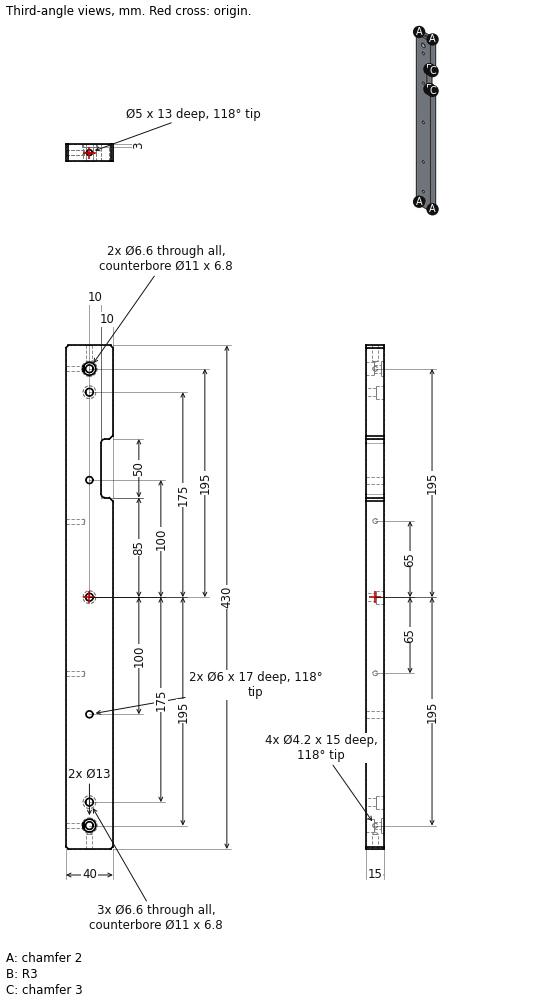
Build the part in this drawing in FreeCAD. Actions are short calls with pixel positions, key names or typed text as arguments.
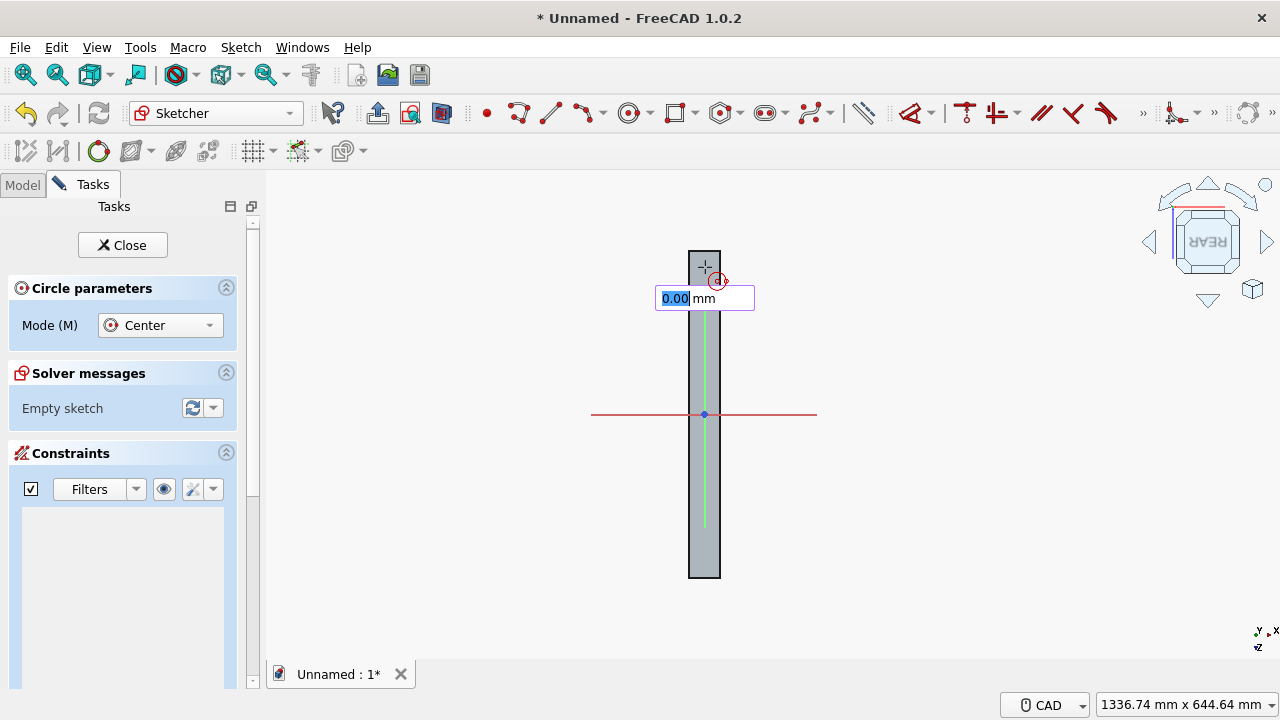
scroll(709, 265, up, 7)
move(708, 264)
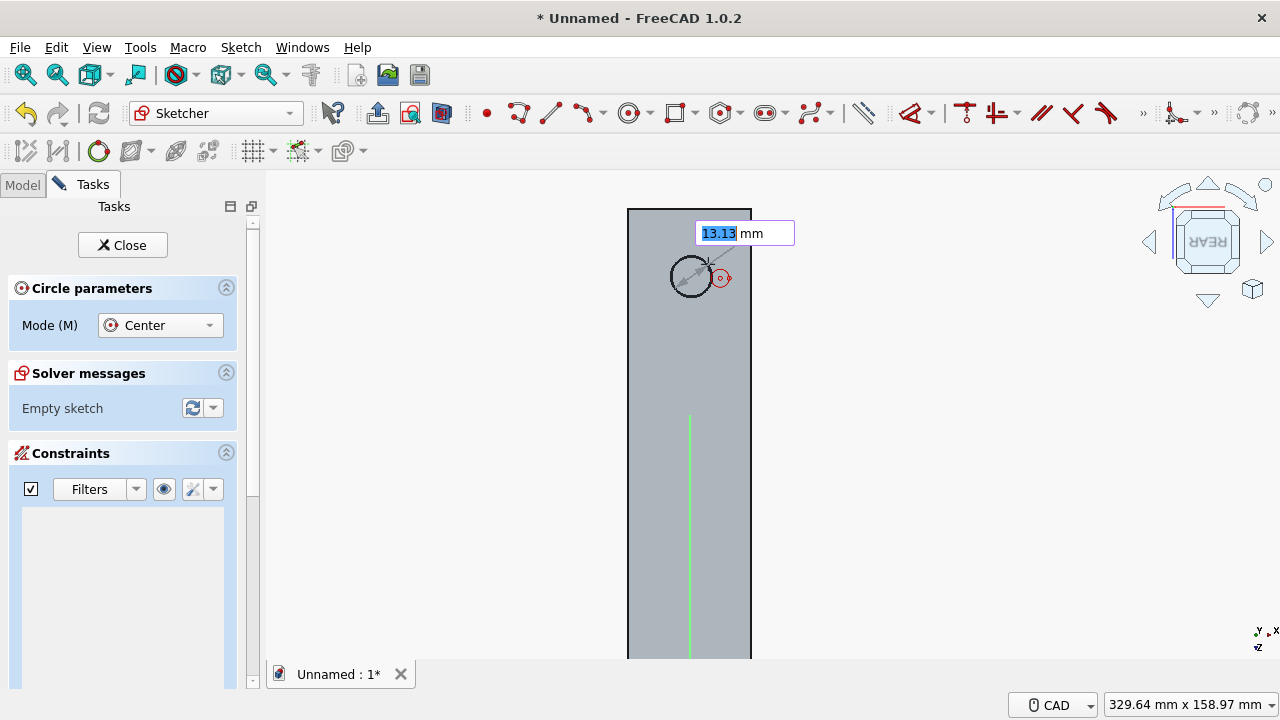
text(13)
key(Return)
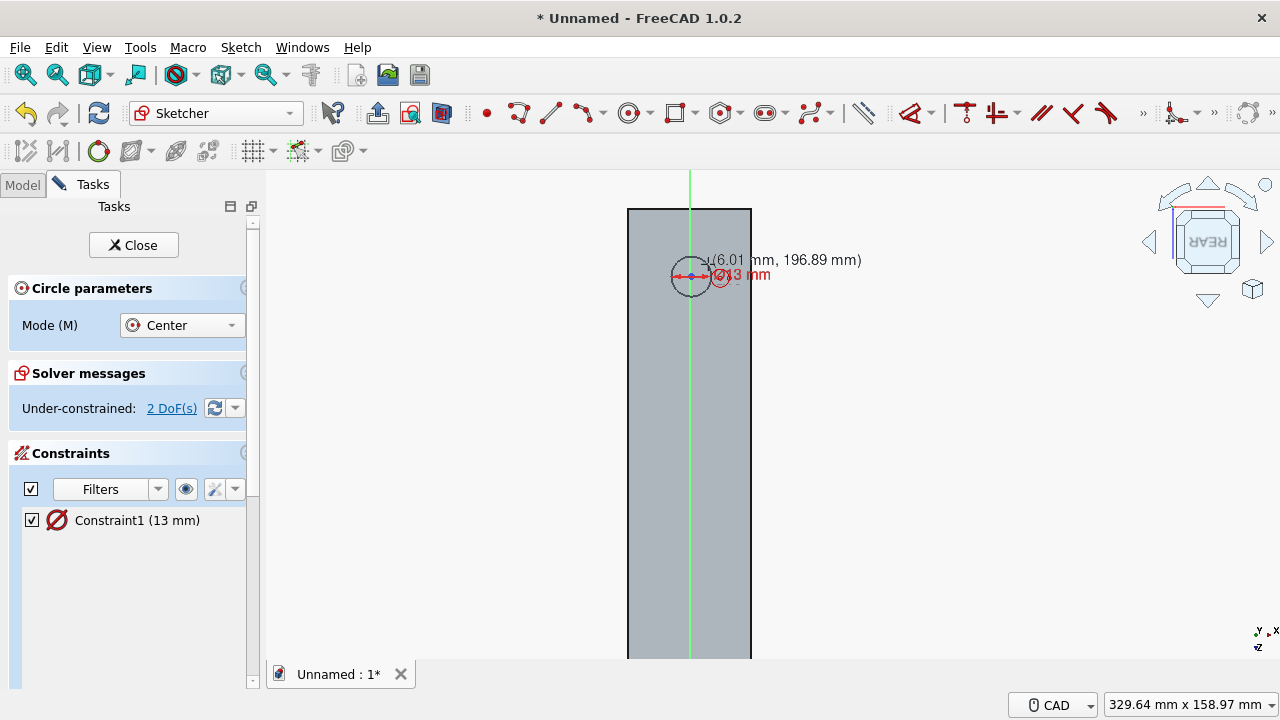
scroll(709, 265, down, 7)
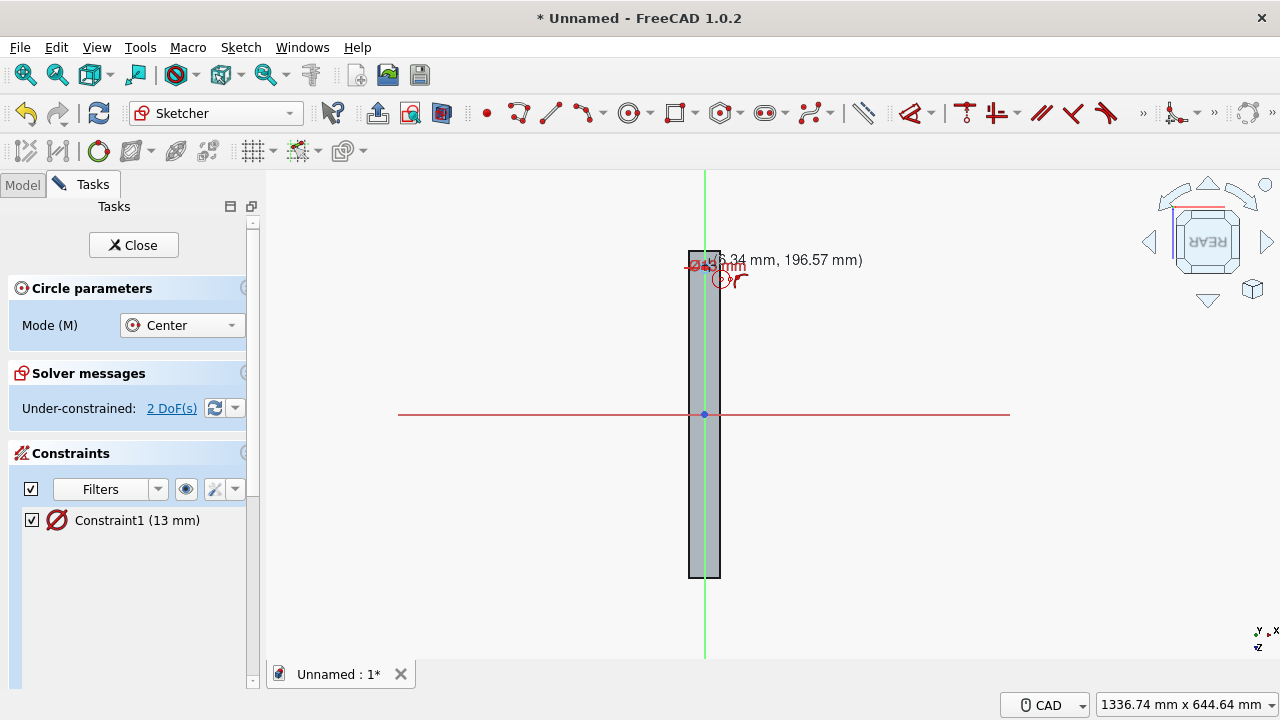
scroll(705, 562, up, 8)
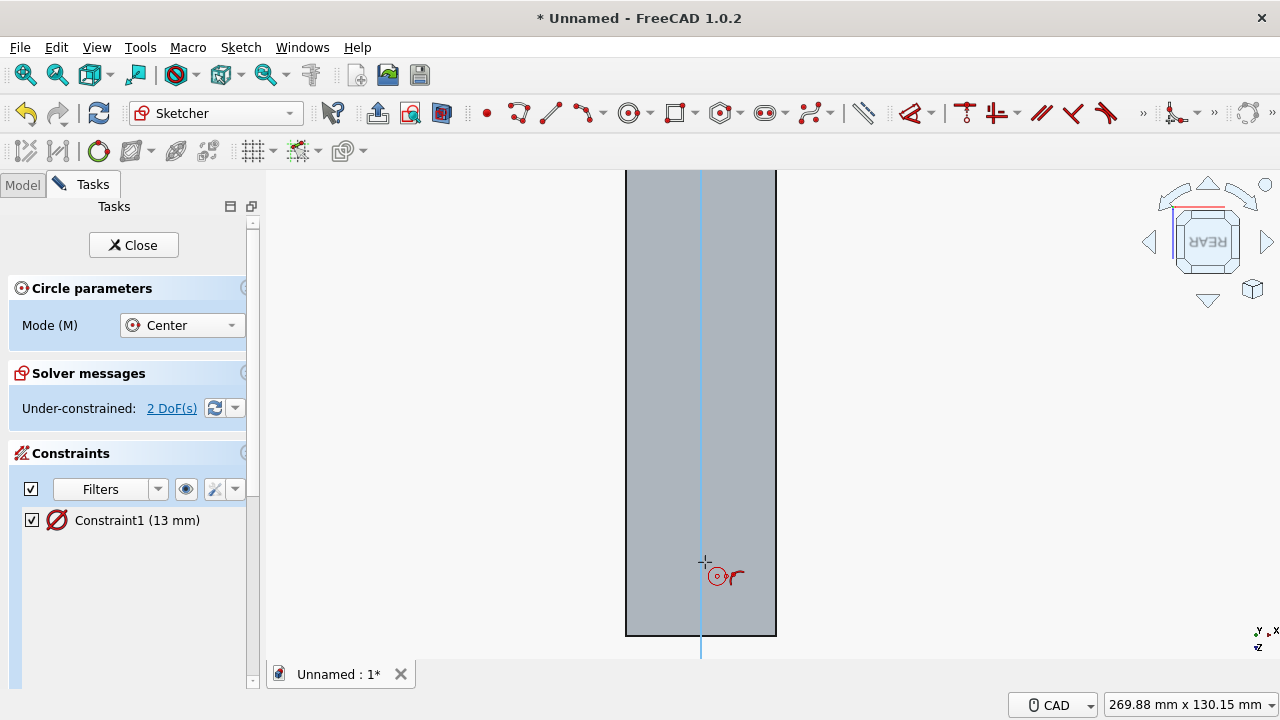
scroll(705, 563, down, 8)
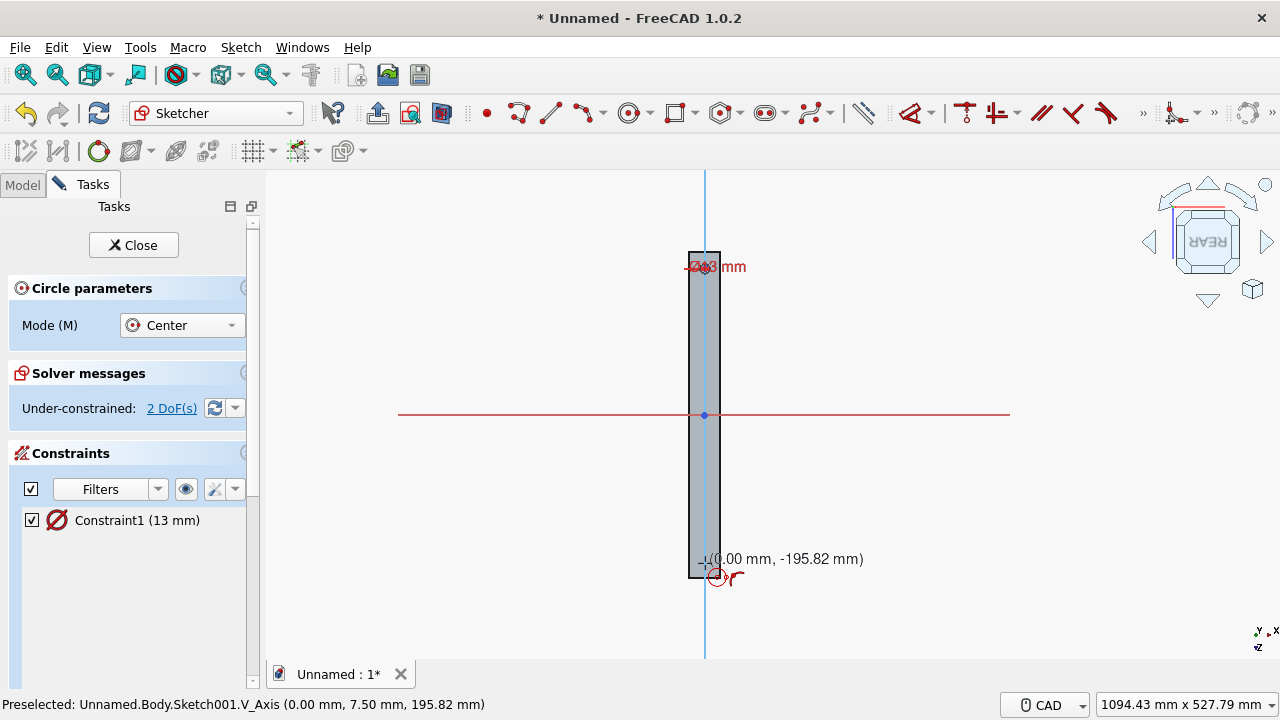
click(705, 563)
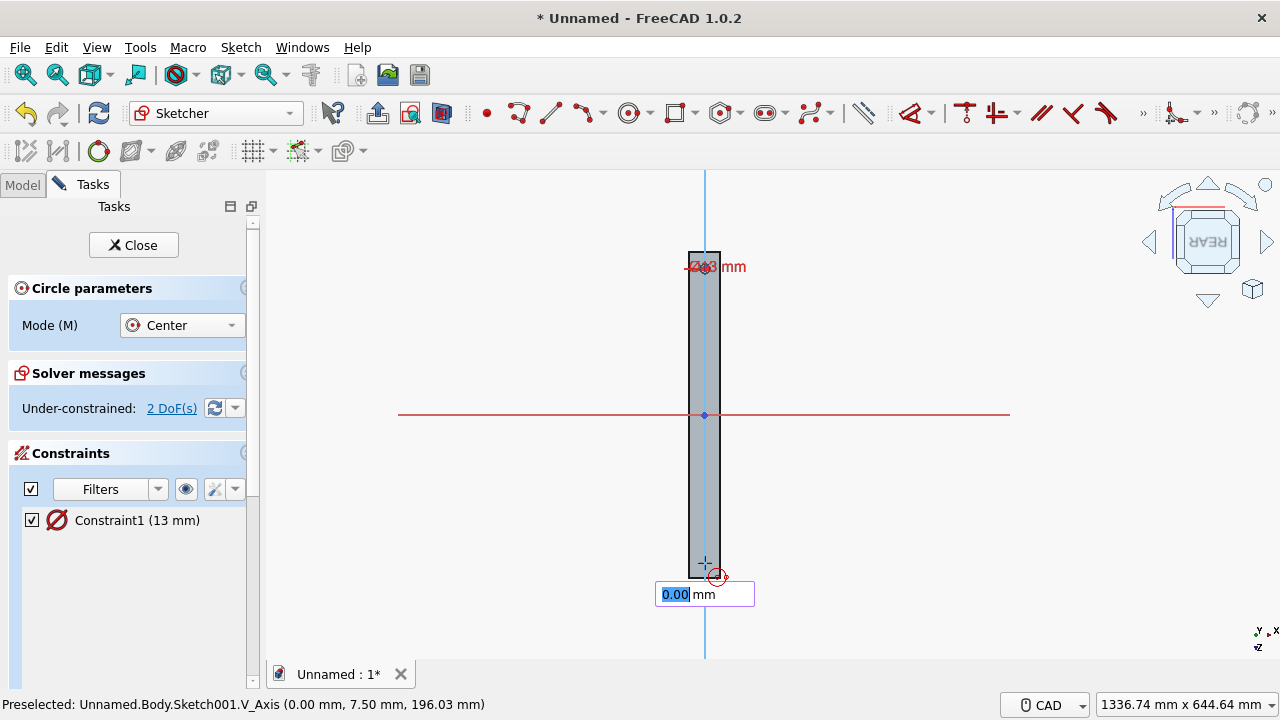
scroll(709, 562, up, 7)
move(708, 558)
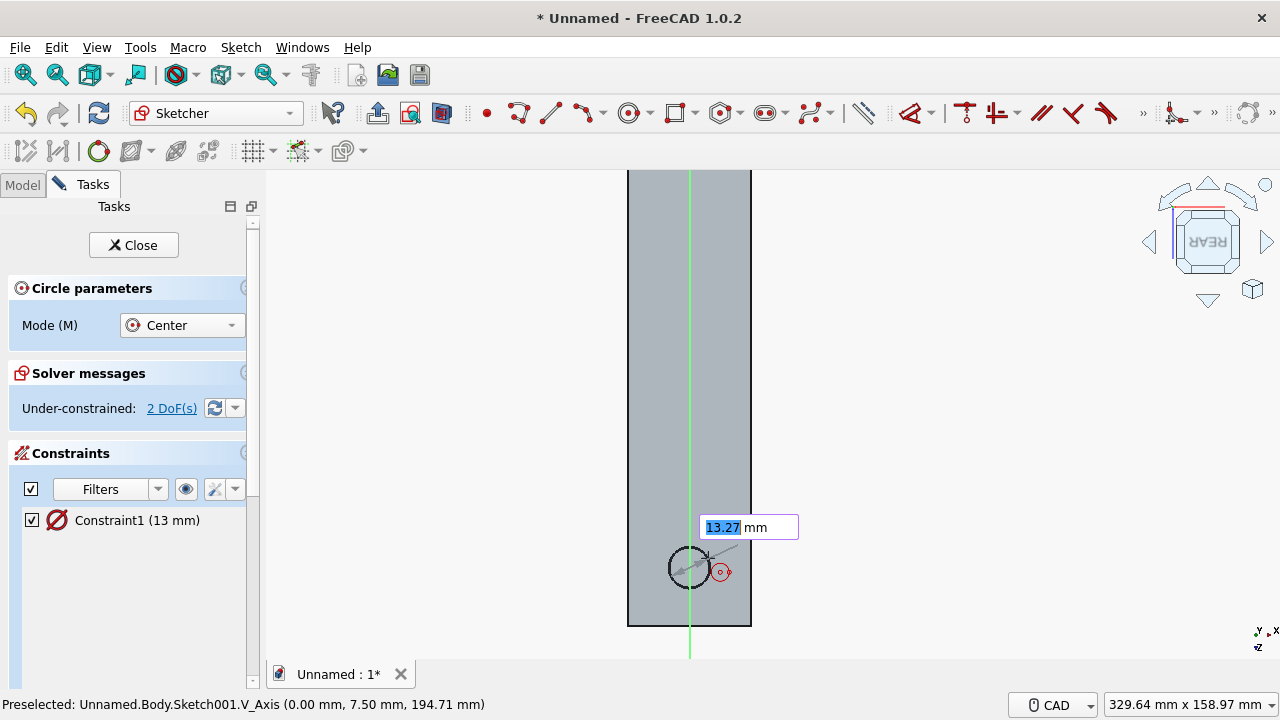
text(13)
key(Return)
key(Escape)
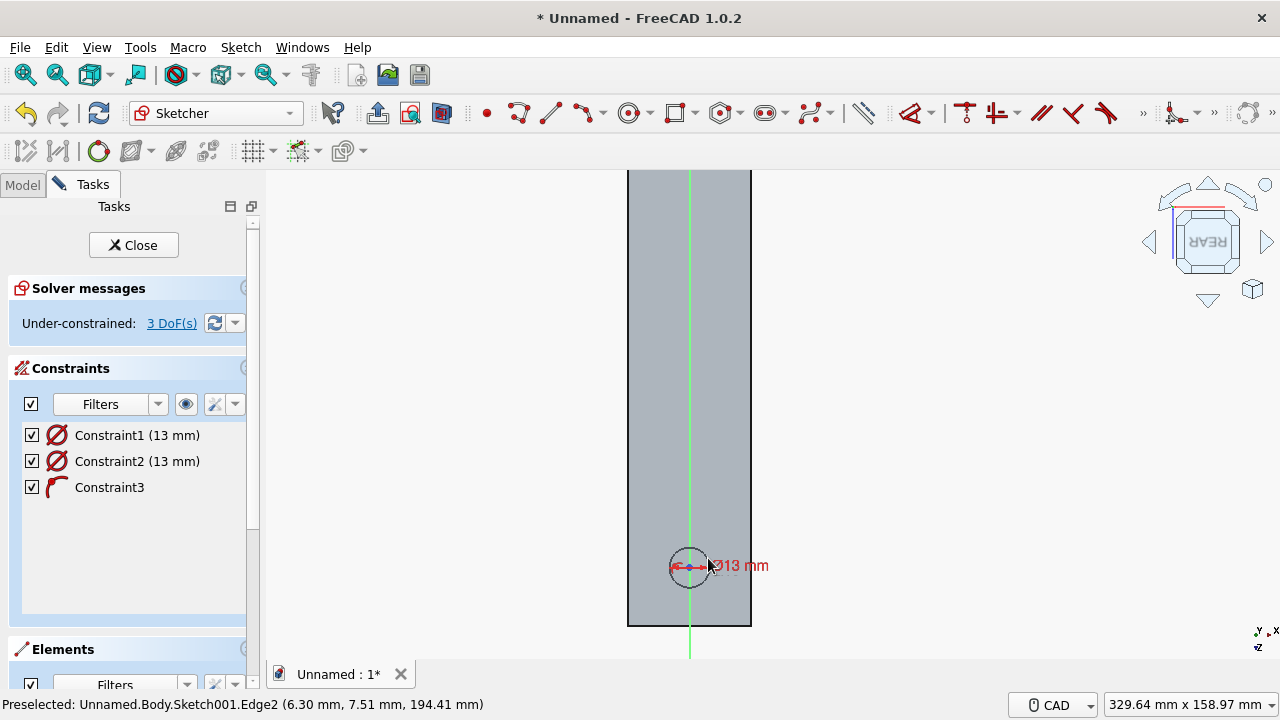
scroll(709, 562, down, 7)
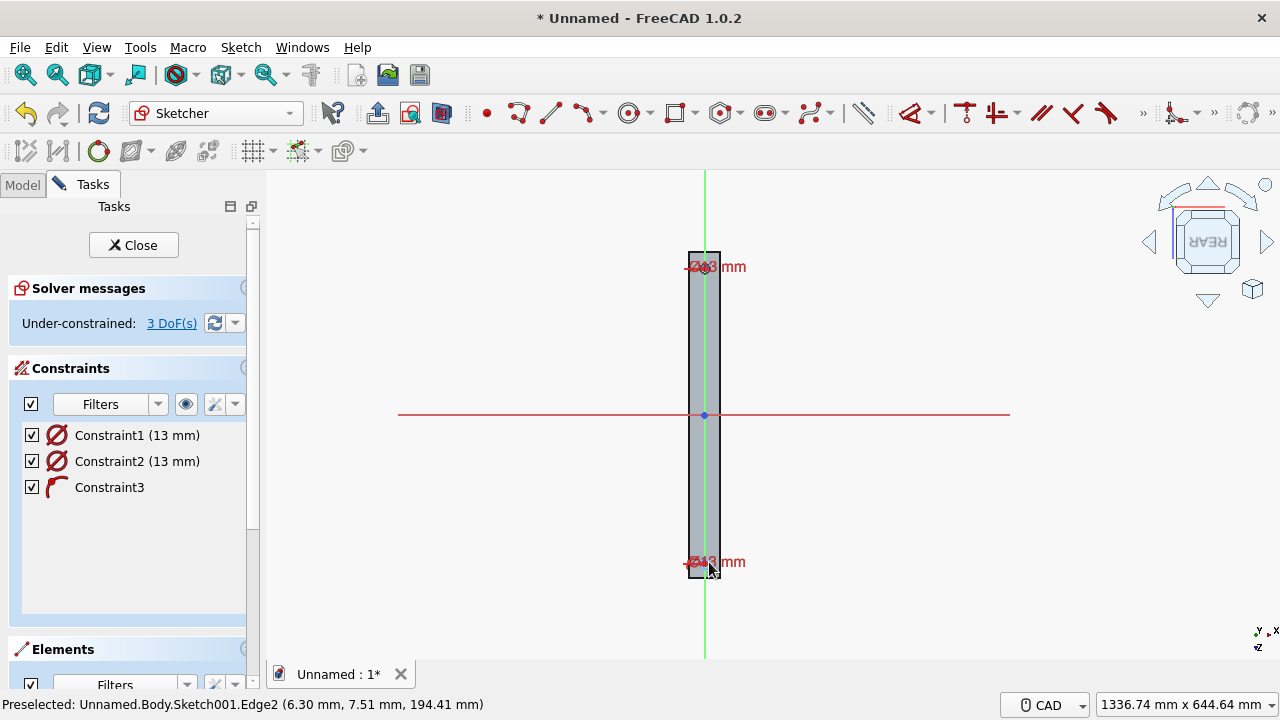
click(705, 269)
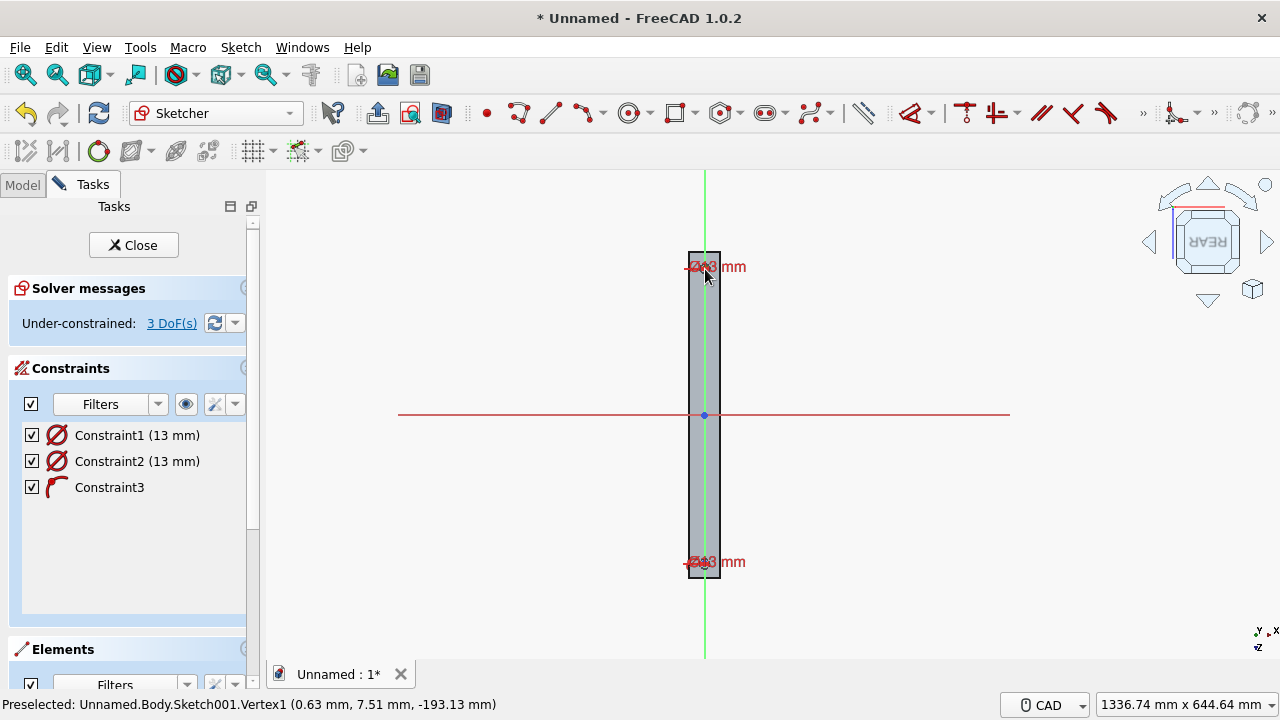
click(705, 600)